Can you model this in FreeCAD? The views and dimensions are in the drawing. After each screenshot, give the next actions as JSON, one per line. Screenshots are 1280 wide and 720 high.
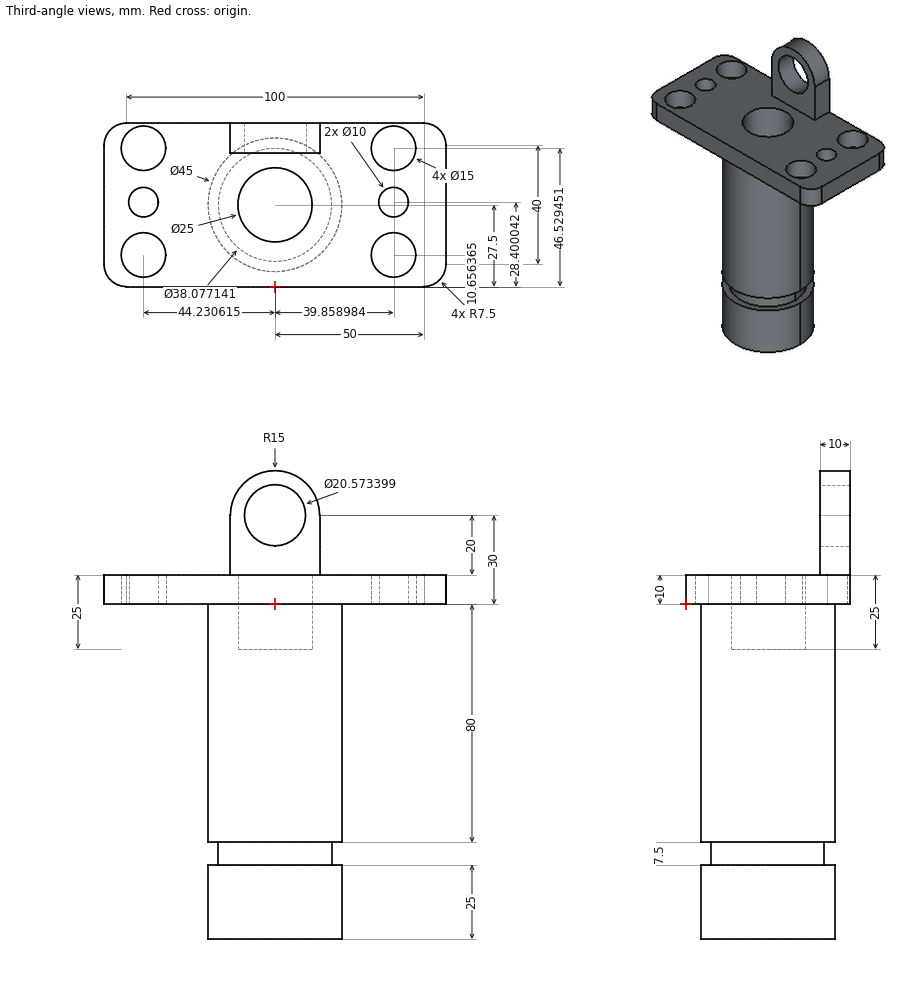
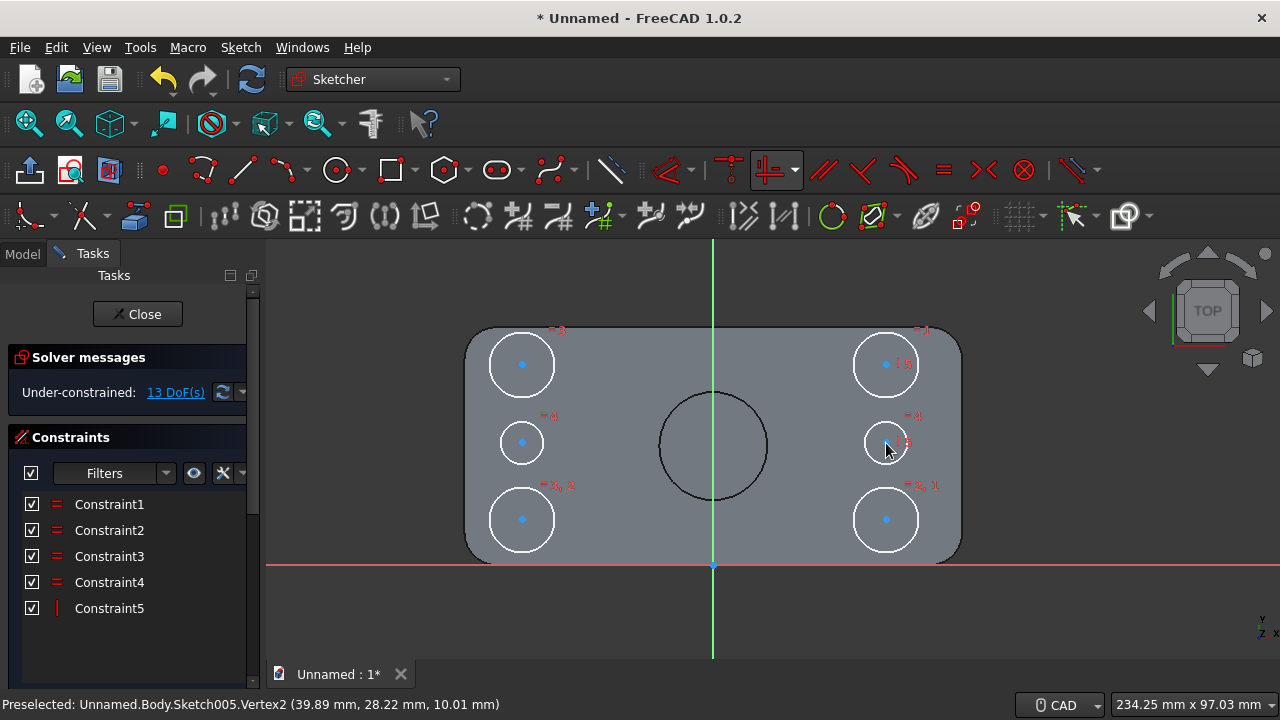
{"action": "left_click", "coordinate": [886, 443]}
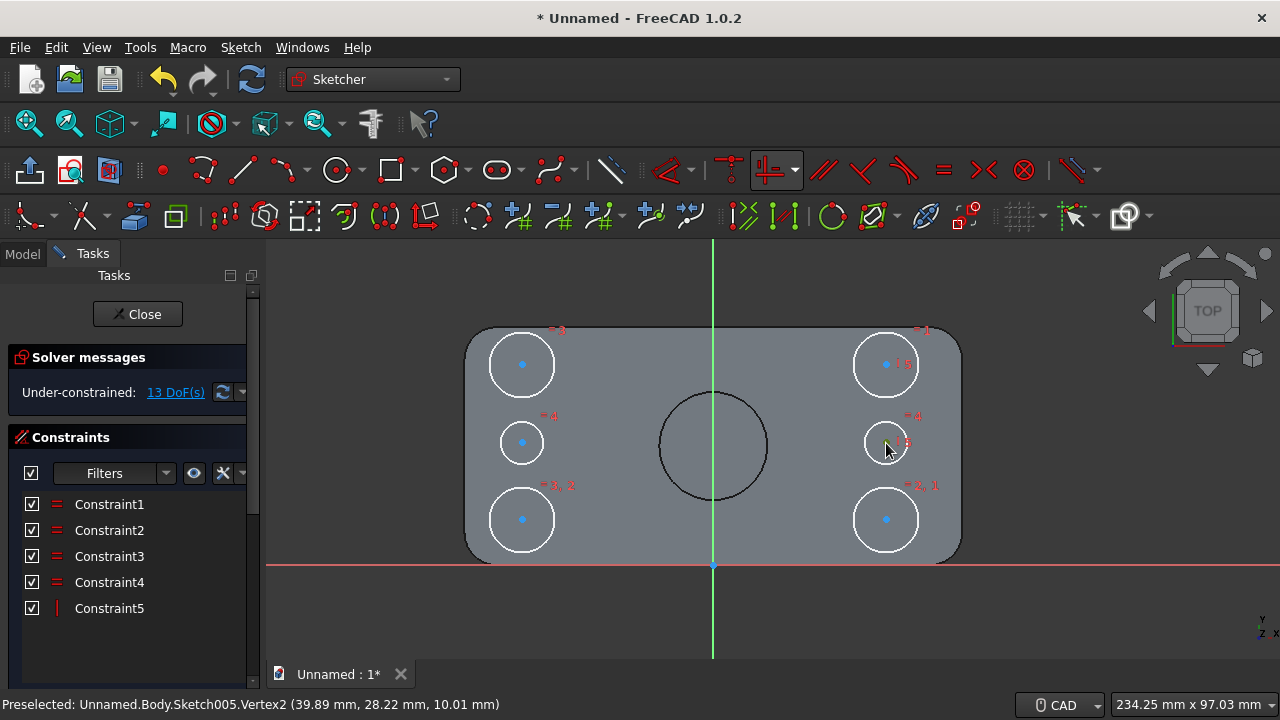
{"action": "left_click", "coordinate": [886, 520]}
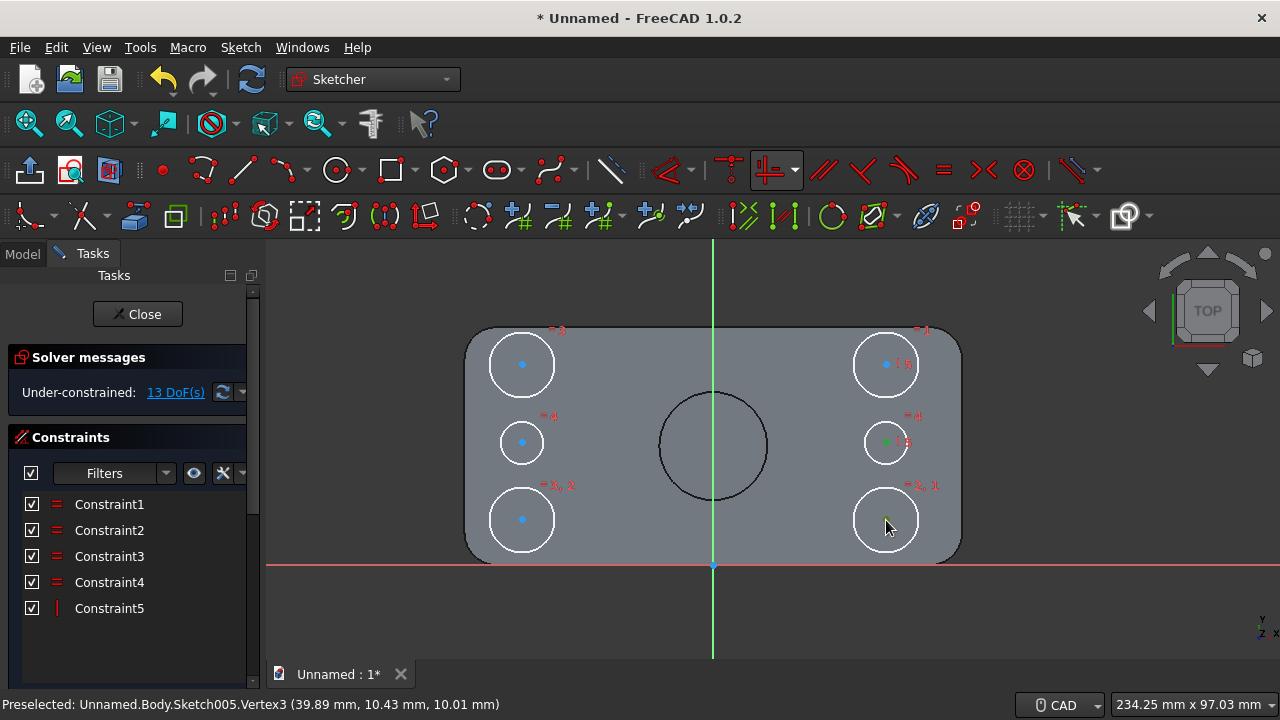
{"action": "left_click", "coordinate": [798, 170]}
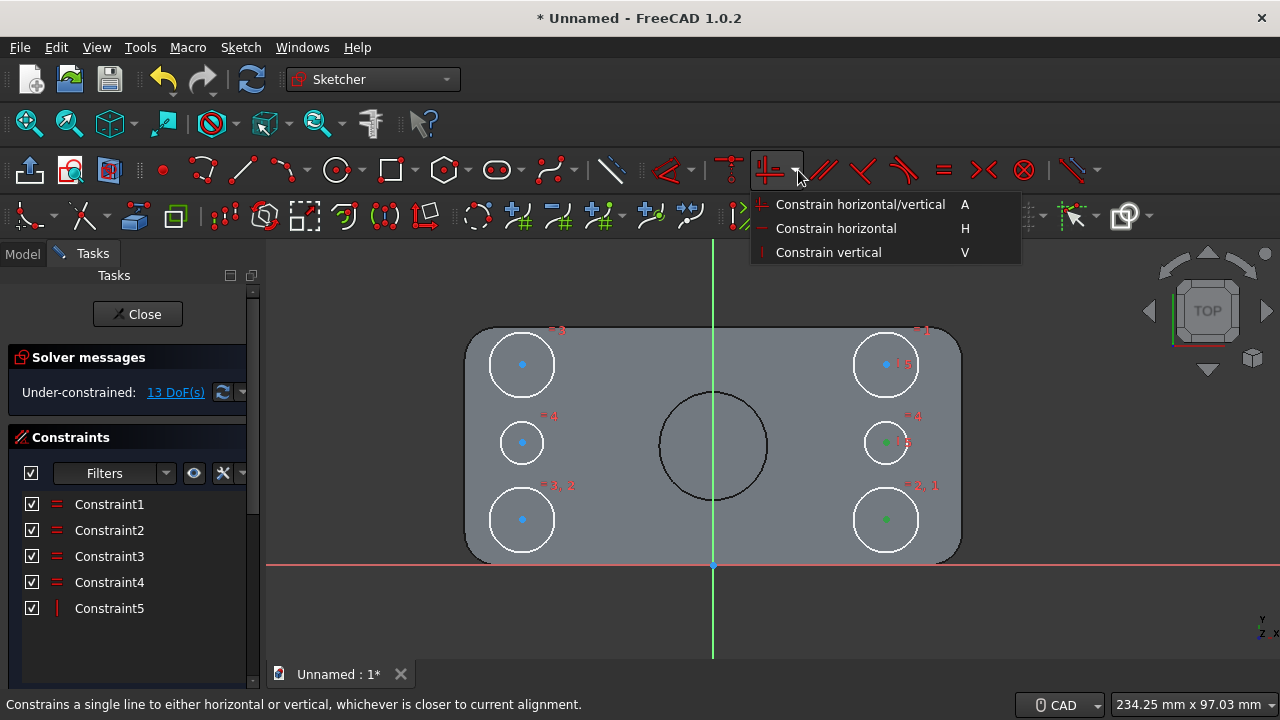
{"action": "left_click", "coordinate": [886, 252]}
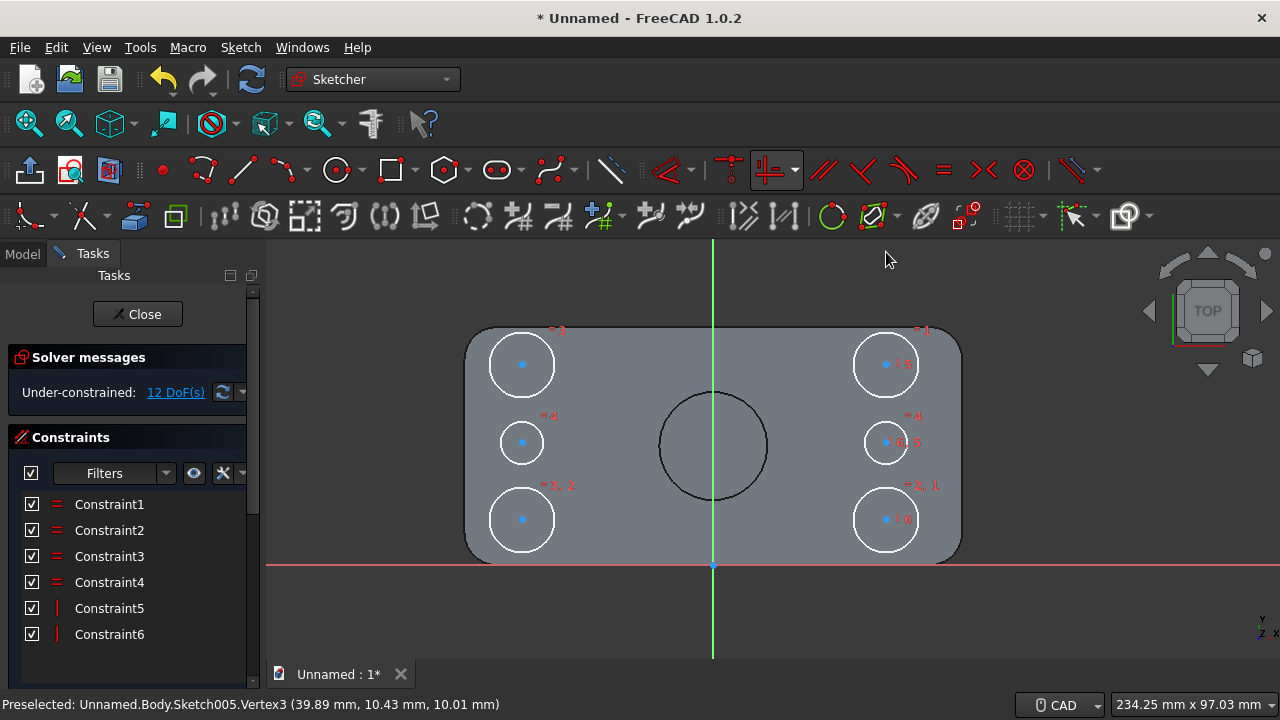
{"action": "left_click", "coordinate": [886, 520]}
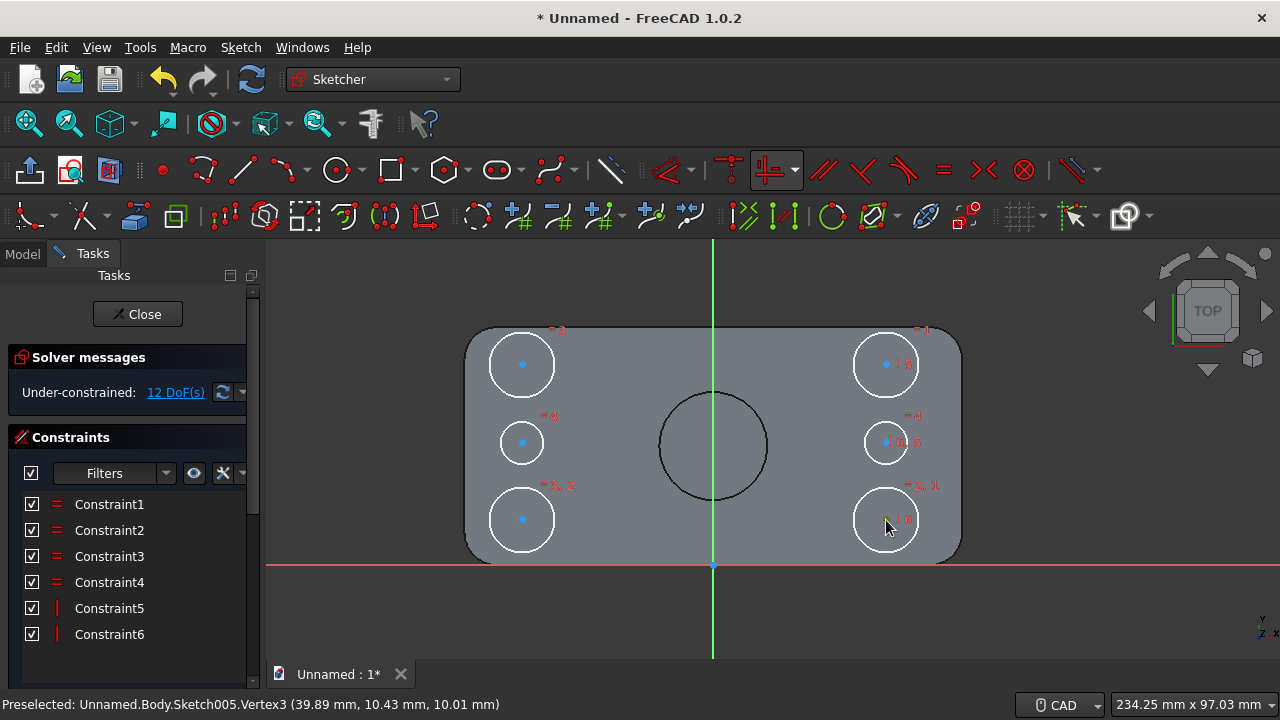
{"action": "left_click", "coordinate": [522, 520]}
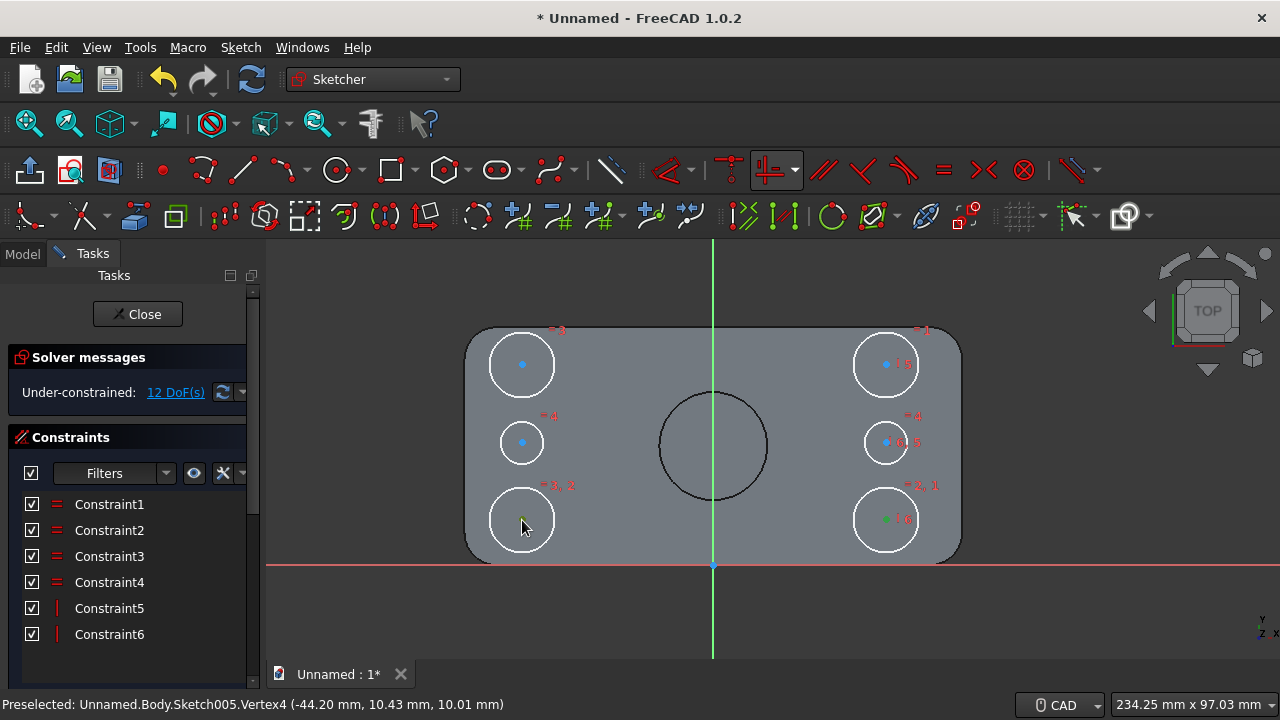
{"action": "left_click", "coordinate": [798, 170]}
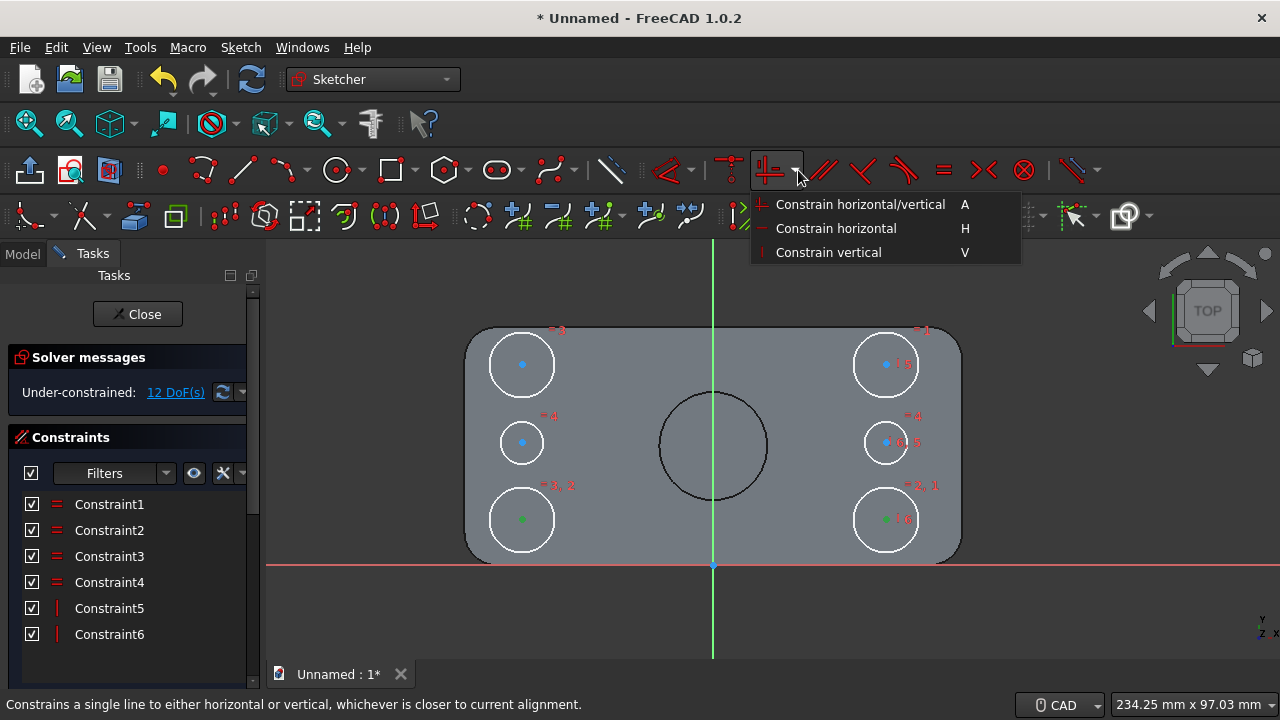
{"action": "left_click", "coordinate": [886, 228]}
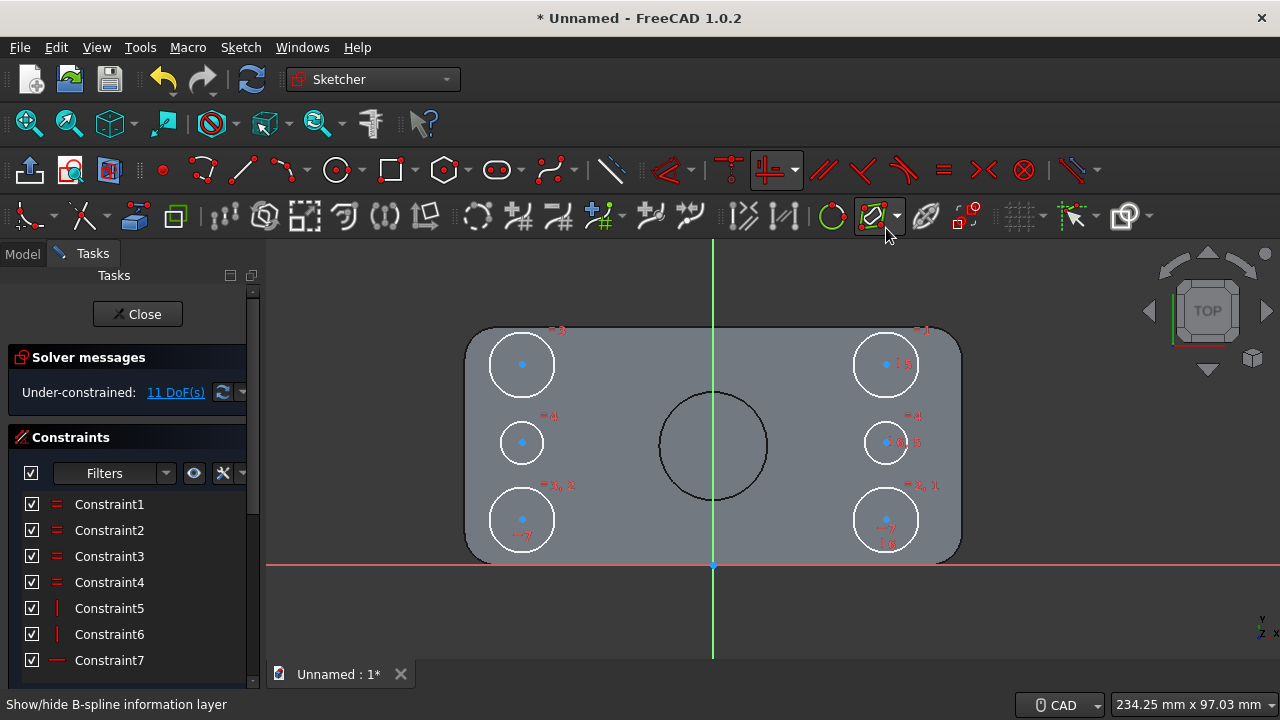
{"action": "left_click", "coordinate": [522, 520]}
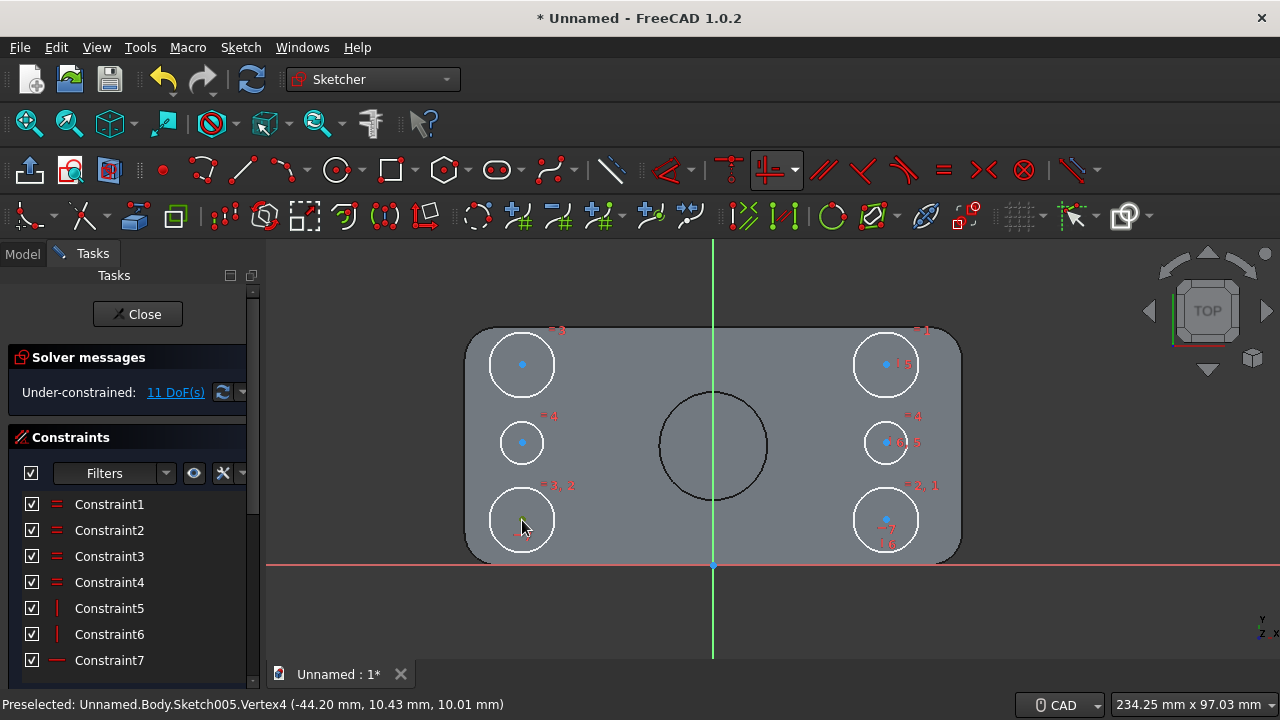
{"action": "left_click", "coordinate": [522, 443]}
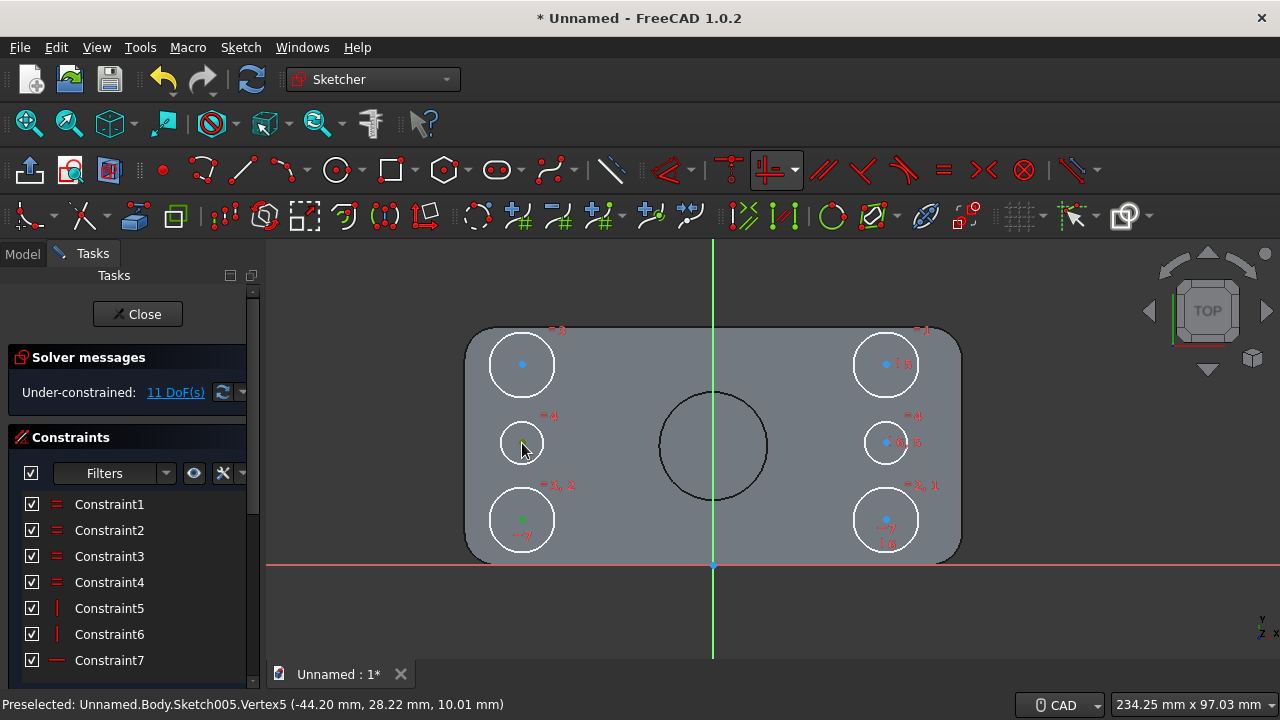
{"action": "key", "text": "v"}